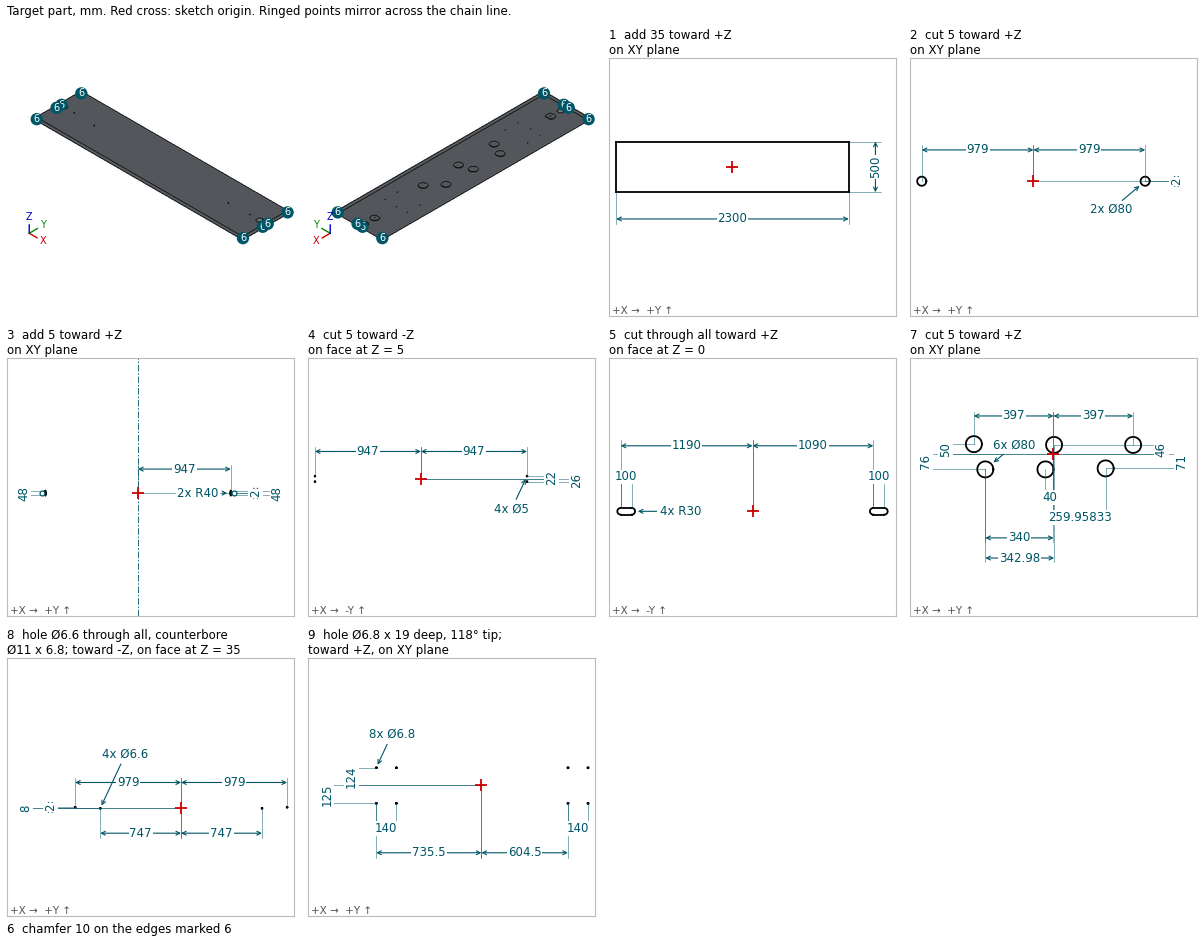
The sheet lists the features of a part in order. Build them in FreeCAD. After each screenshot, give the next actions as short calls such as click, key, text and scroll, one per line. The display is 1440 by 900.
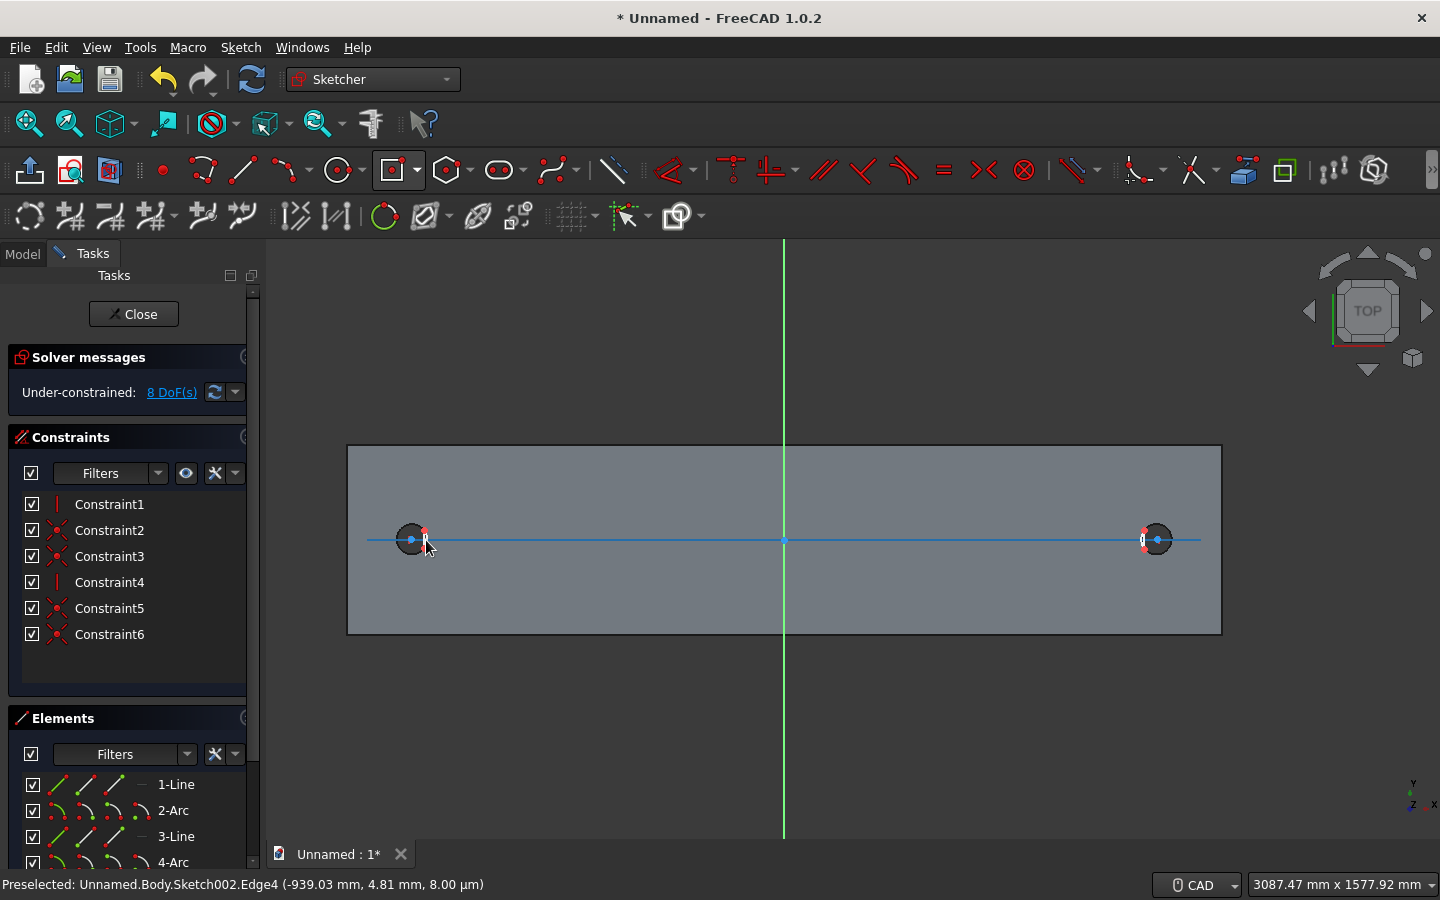
scroll(1142, 536, up, 9)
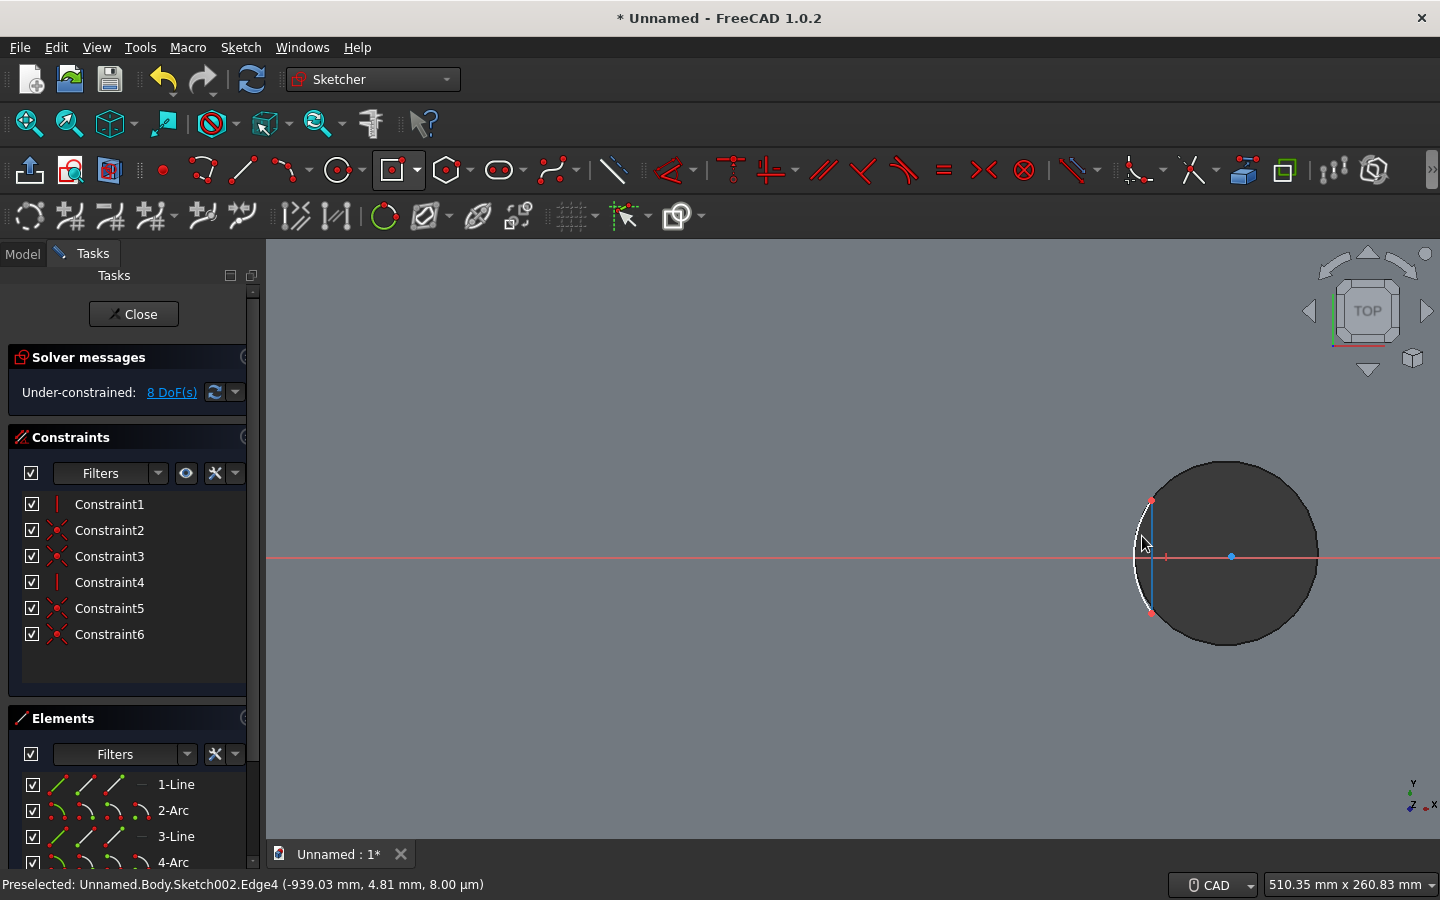
click(1137, 533)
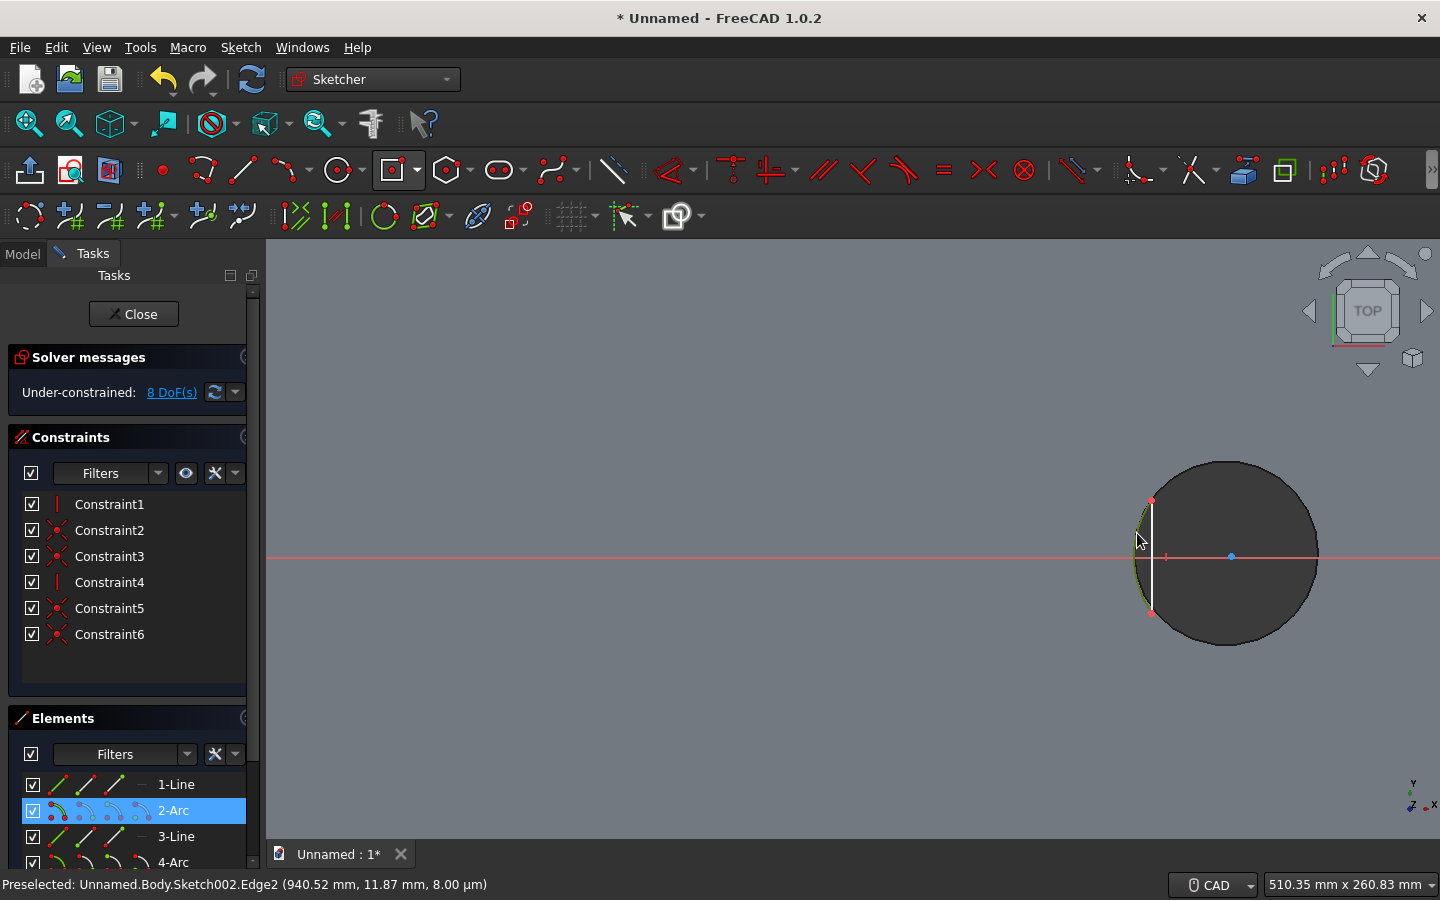
scroll(1143, 536, down, 9)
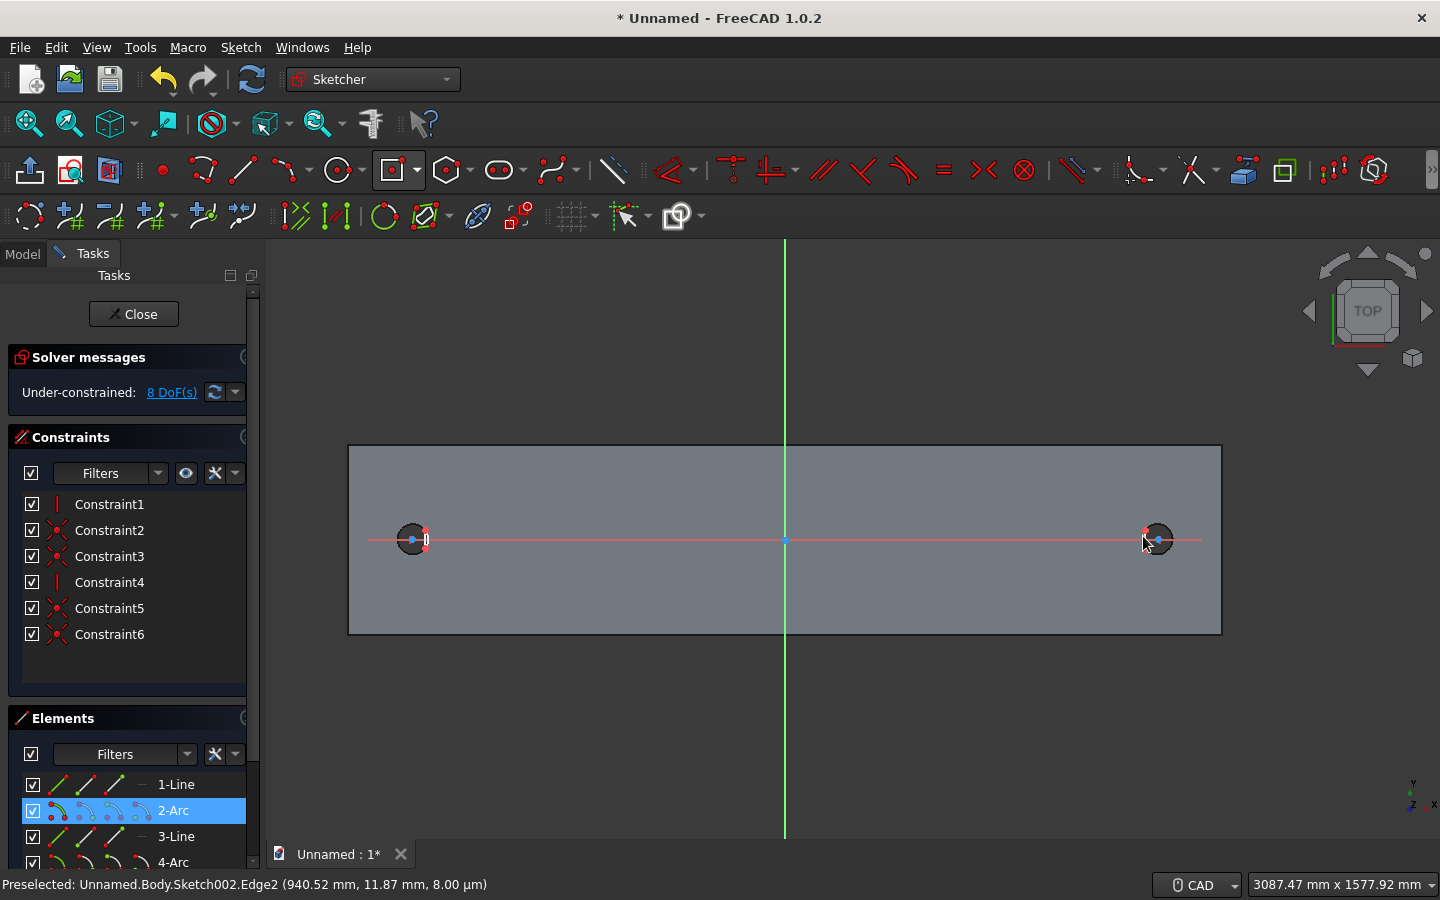
scroll(428, 544, up, 9)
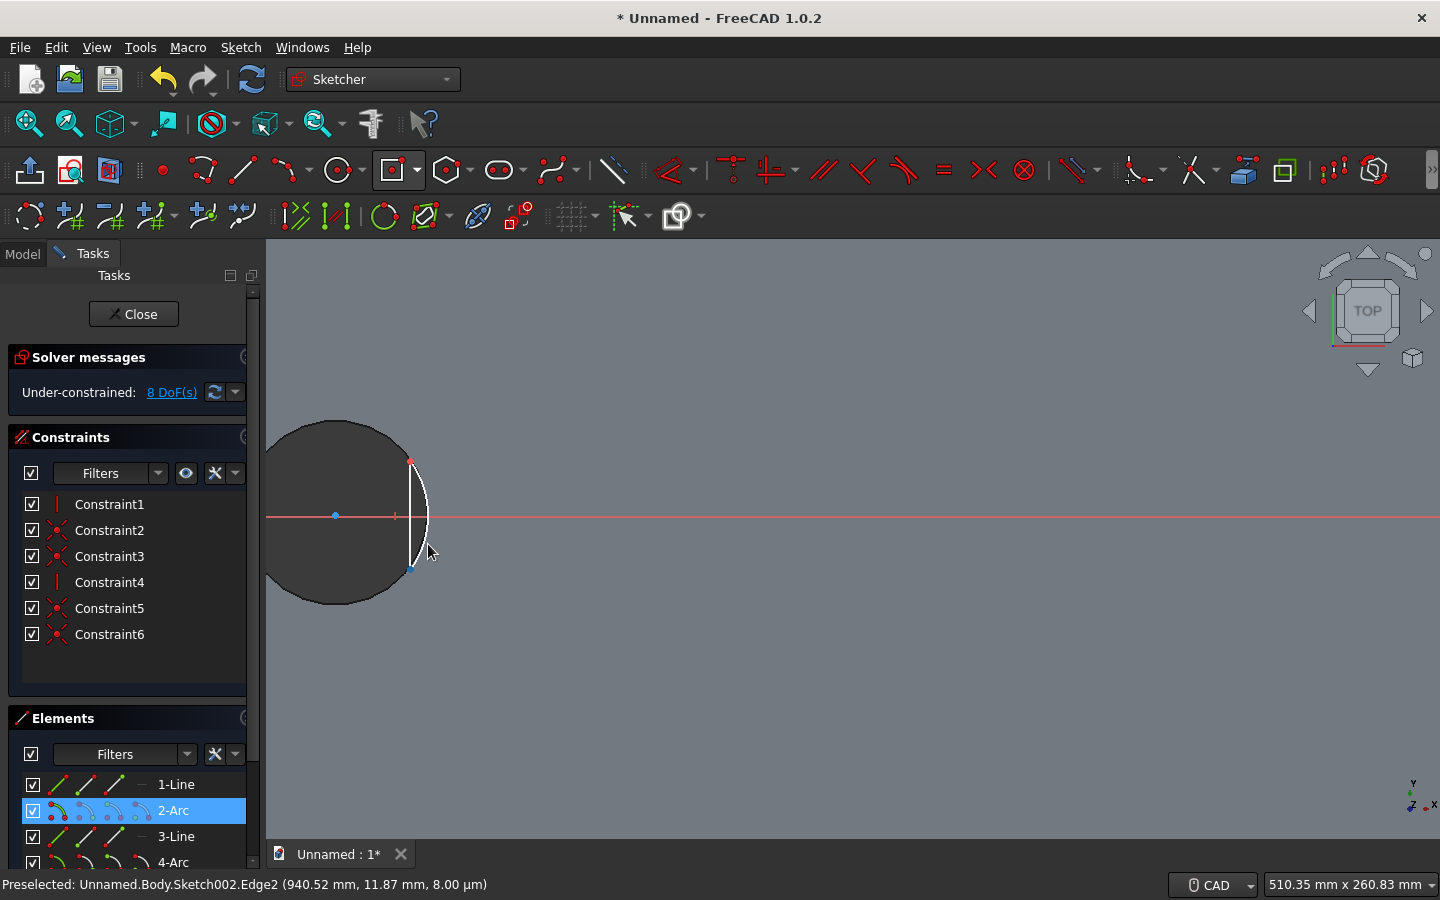
click(425, 539)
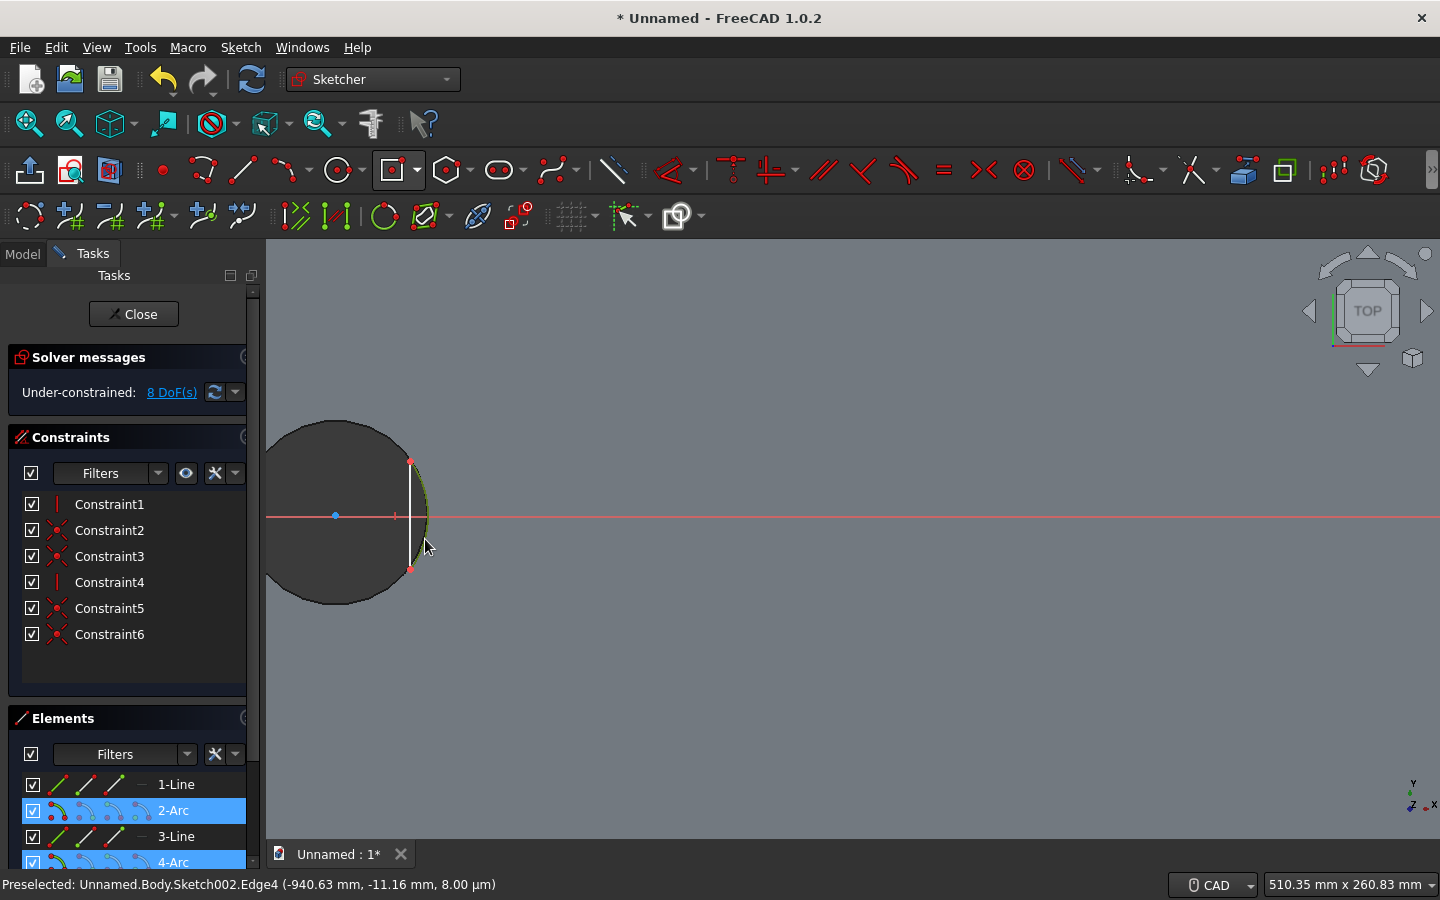
click(944, 170)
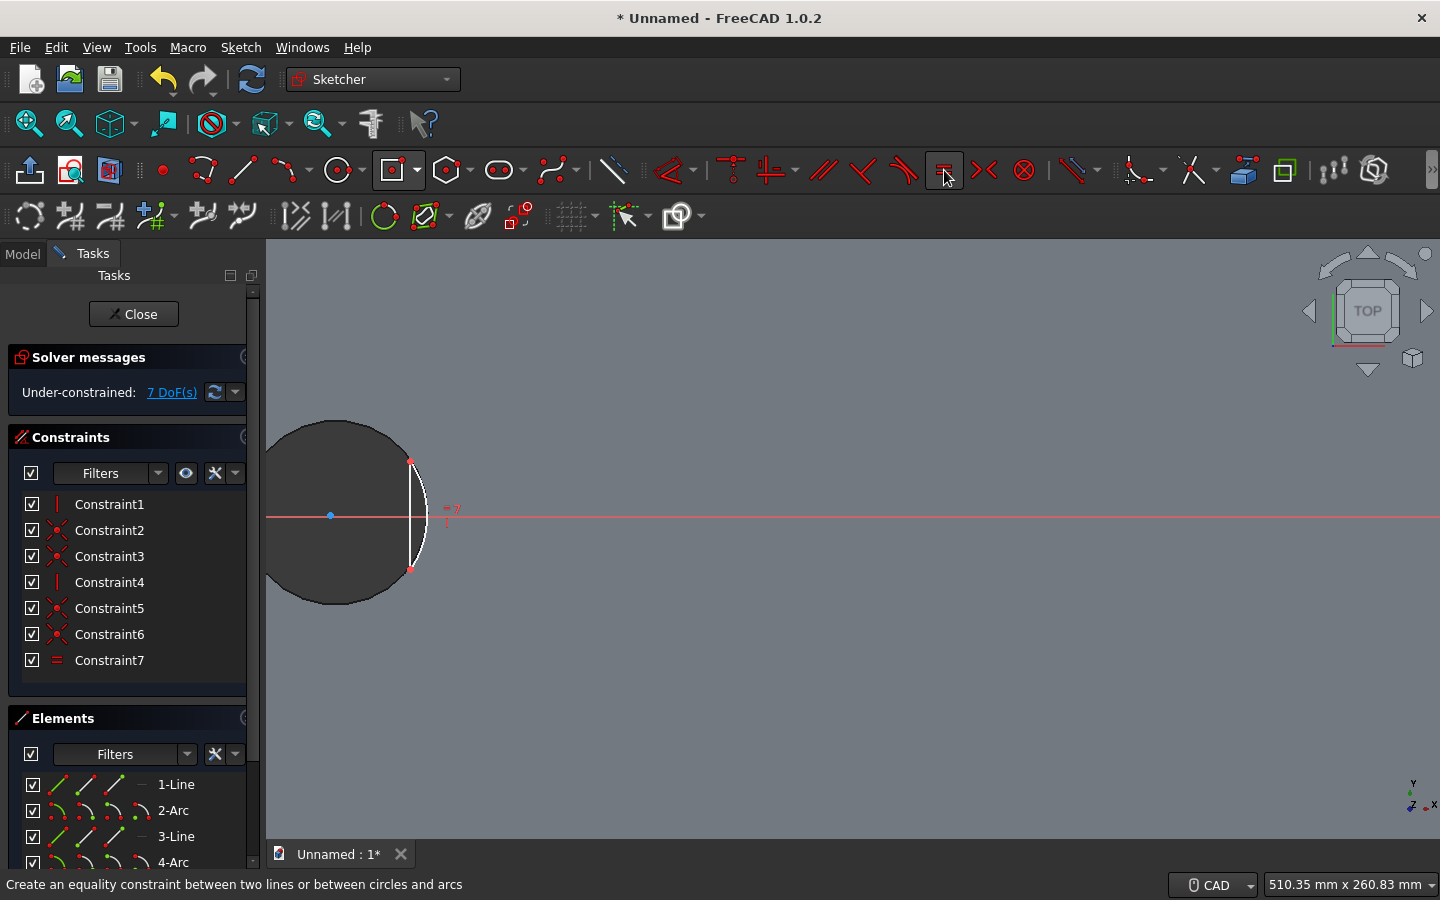
scroll(427, 544, down, 9)